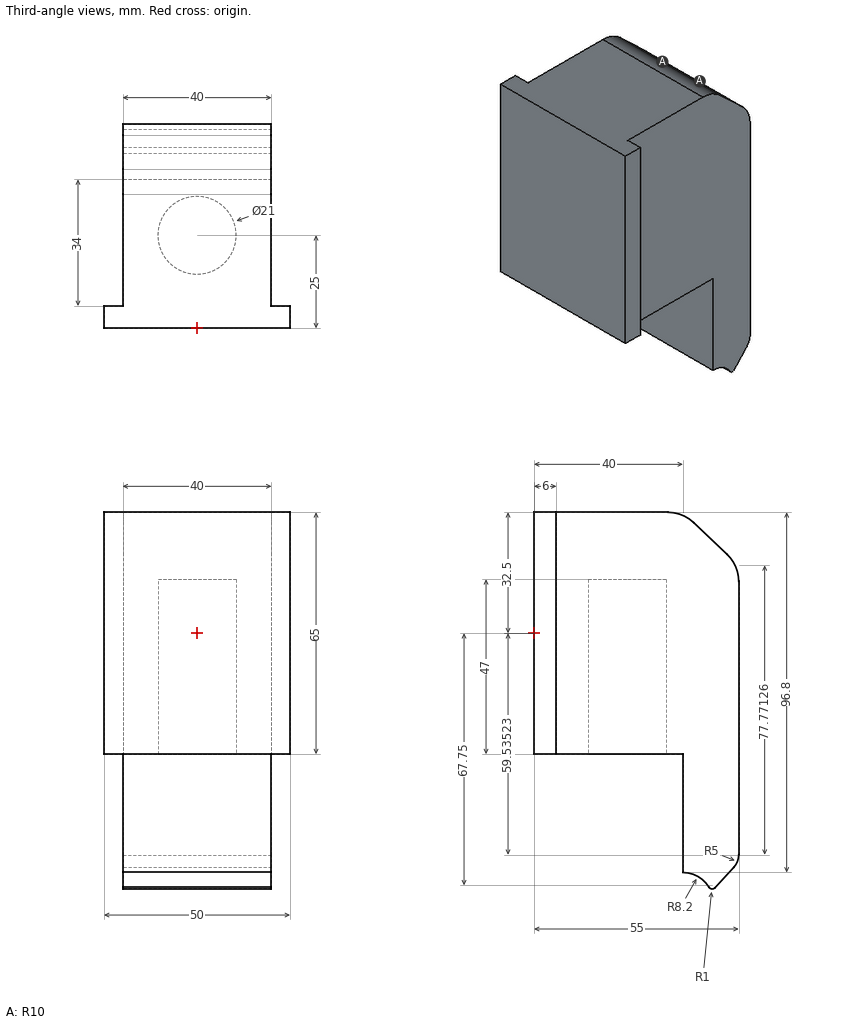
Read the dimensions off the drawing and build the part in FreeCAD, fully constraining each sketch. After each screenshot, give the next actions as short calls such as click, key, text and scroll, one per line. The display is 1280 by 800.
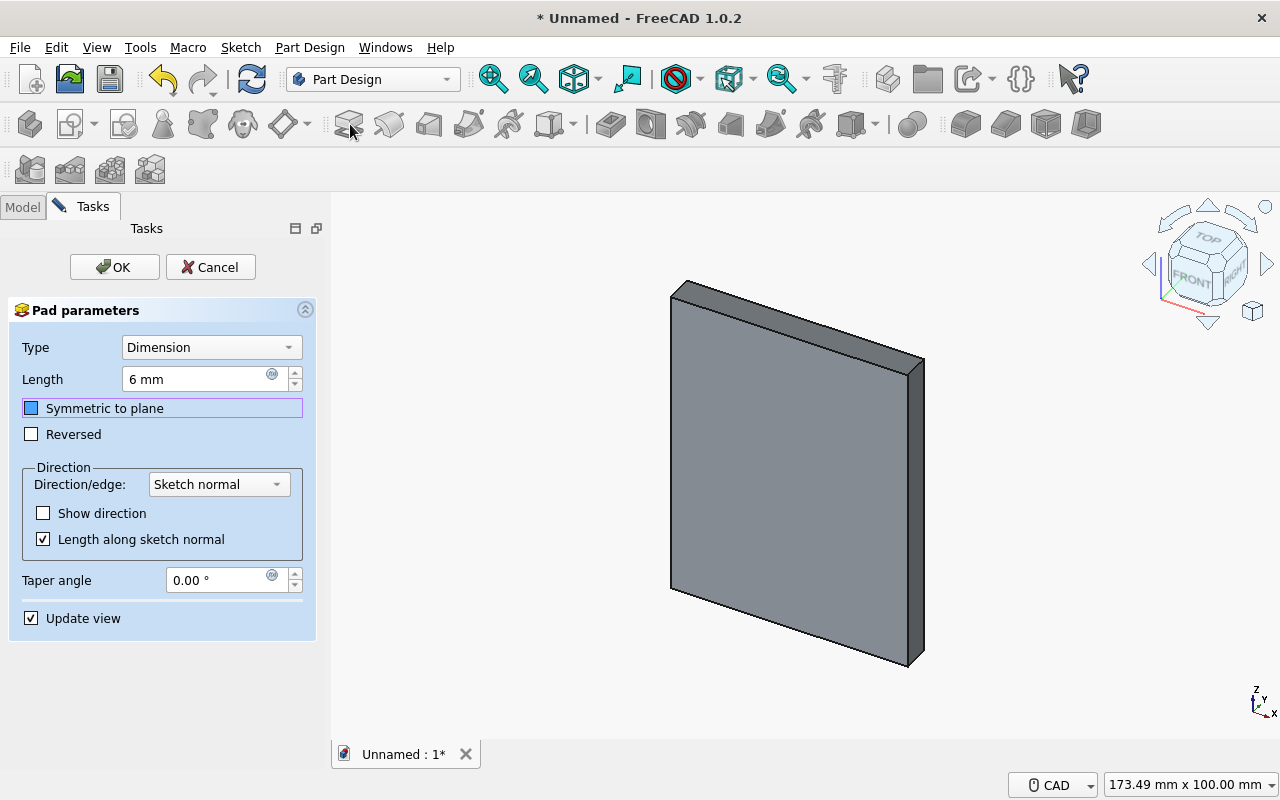
click(30, 434)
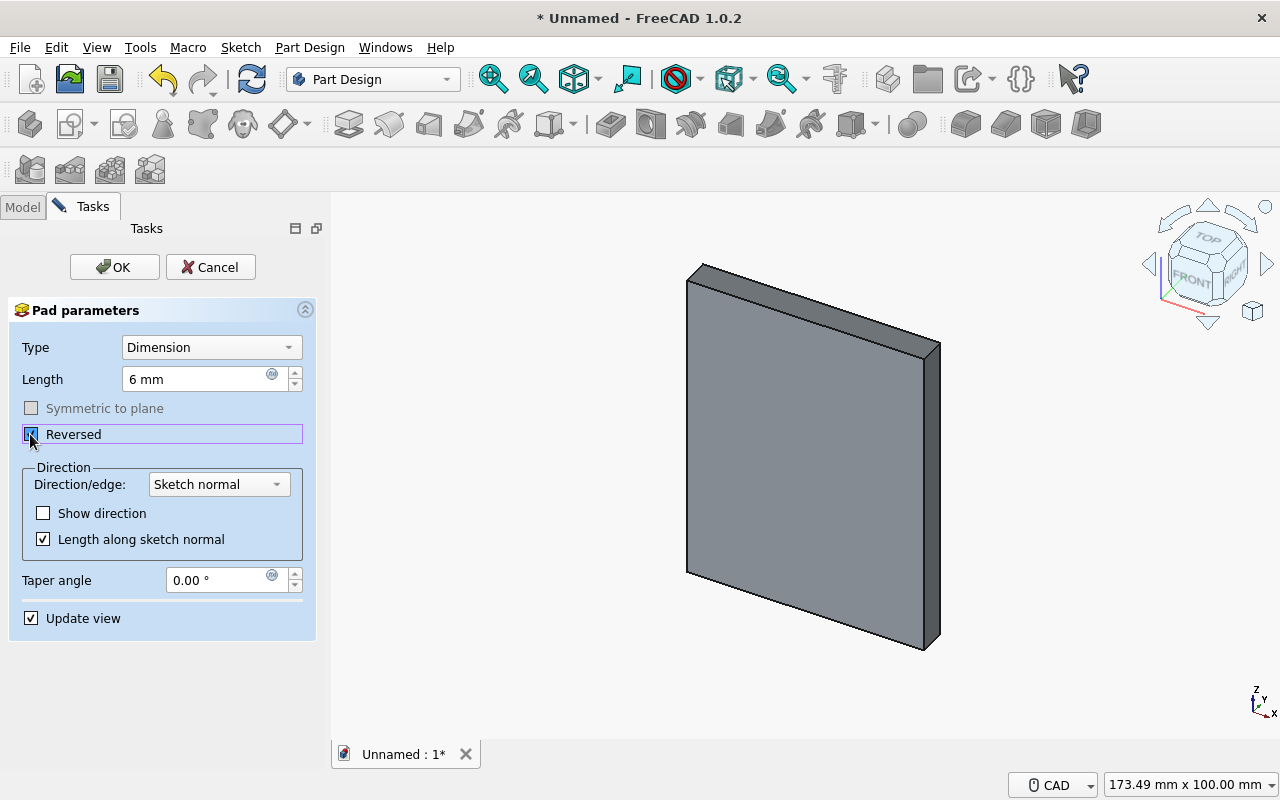
click(115, 267)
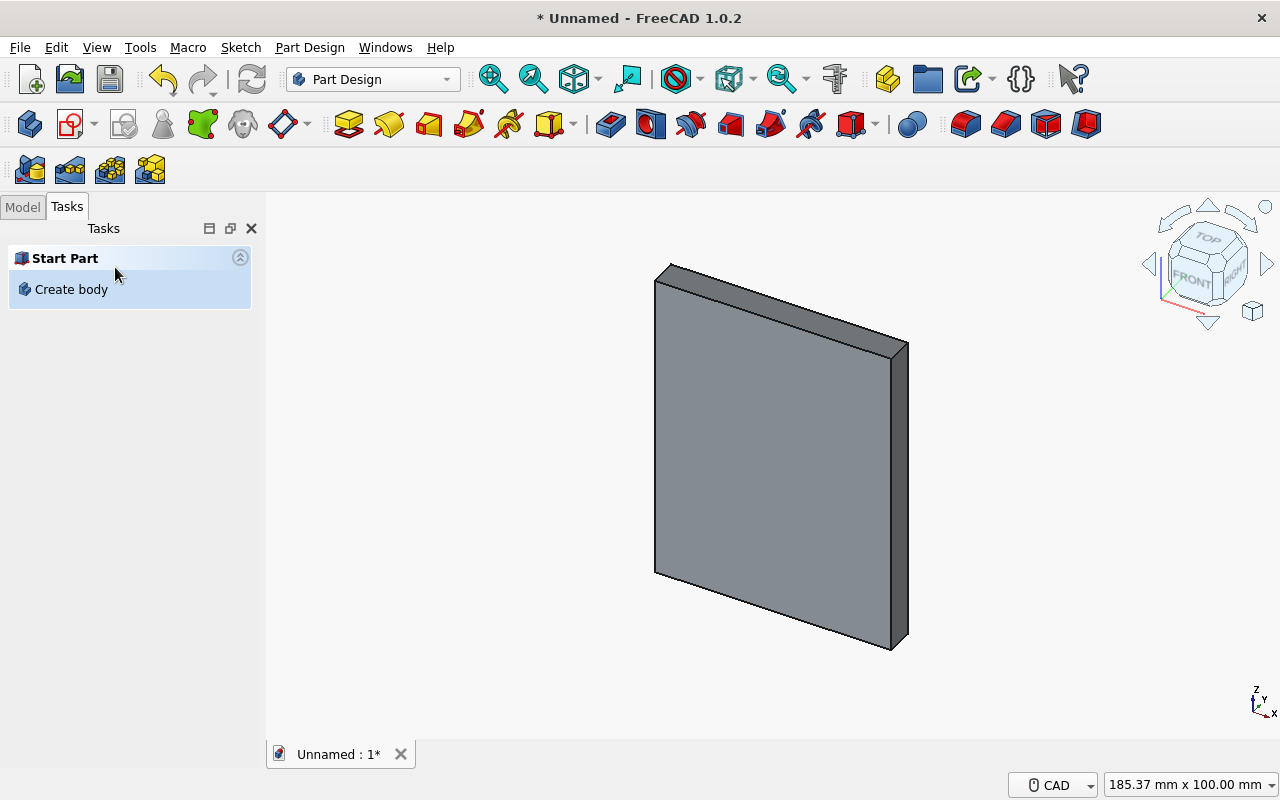
key(4)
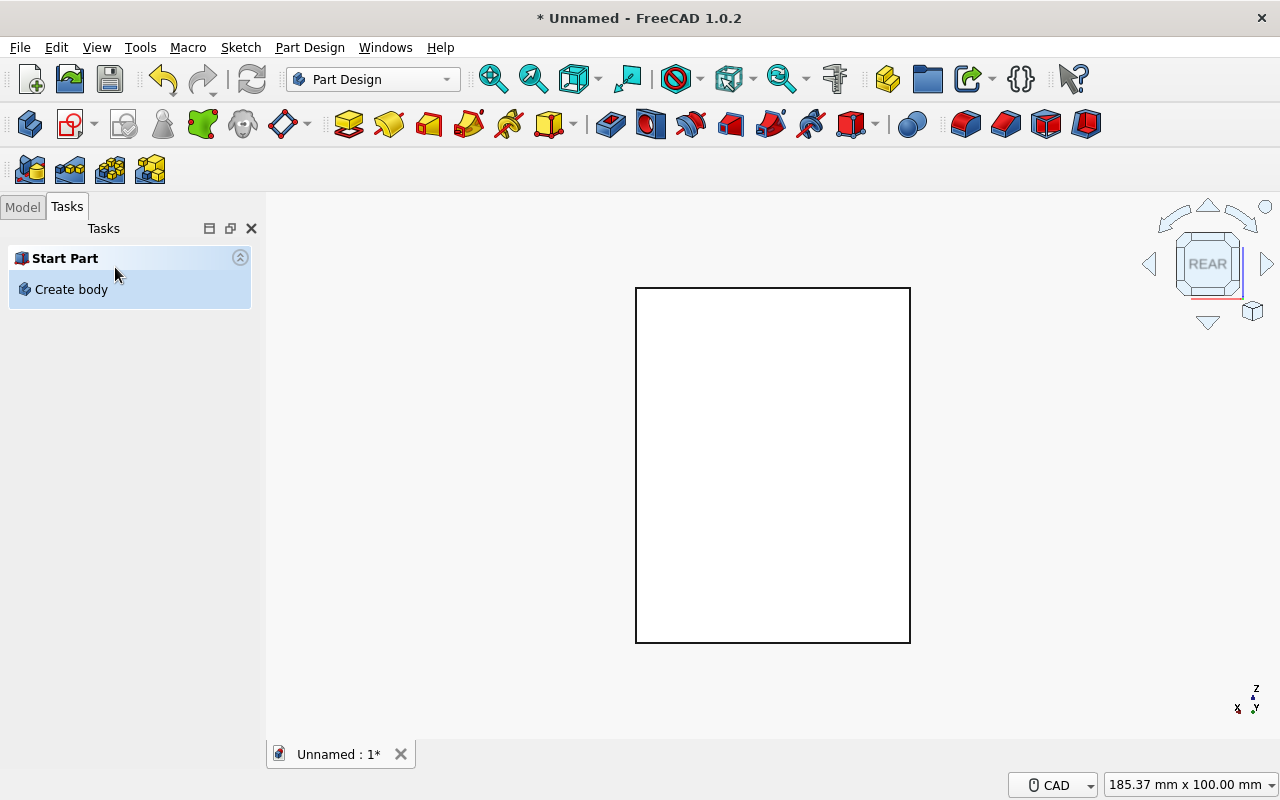
click(773, 464)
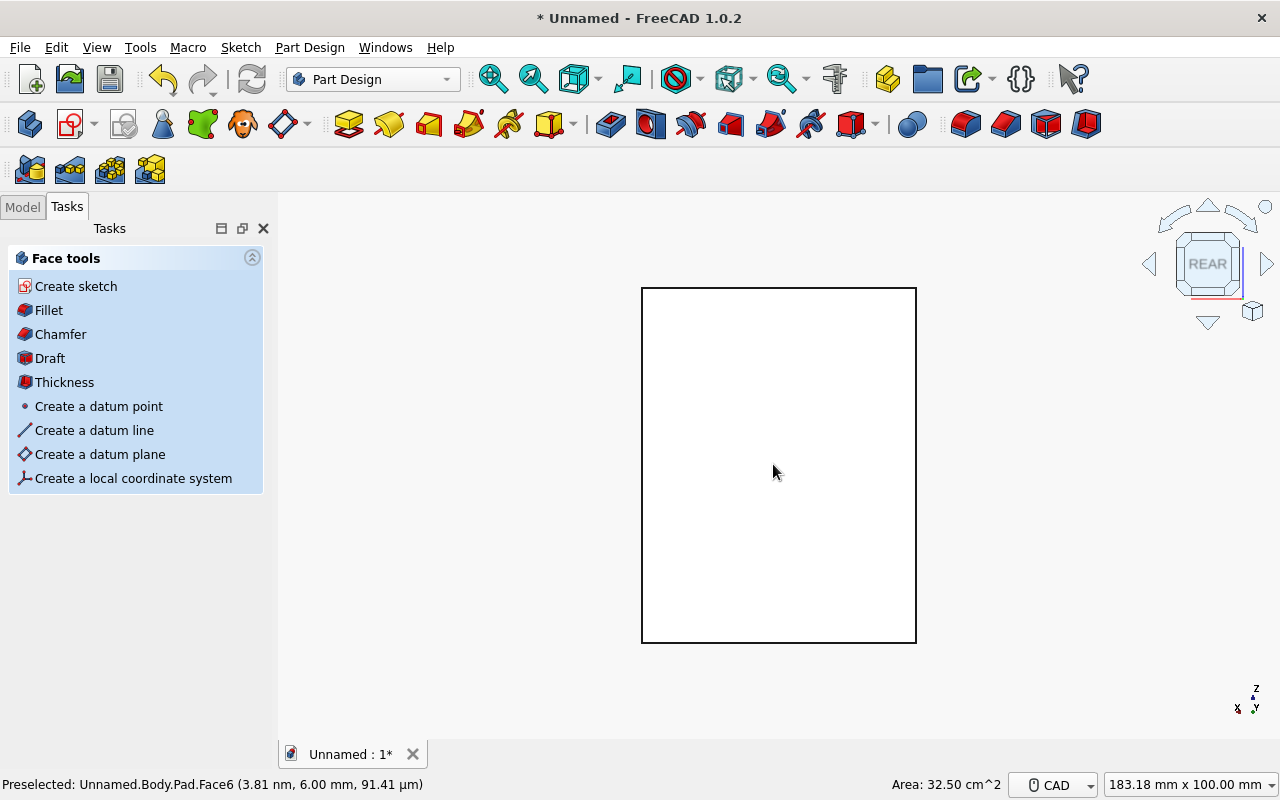
click(70, 124)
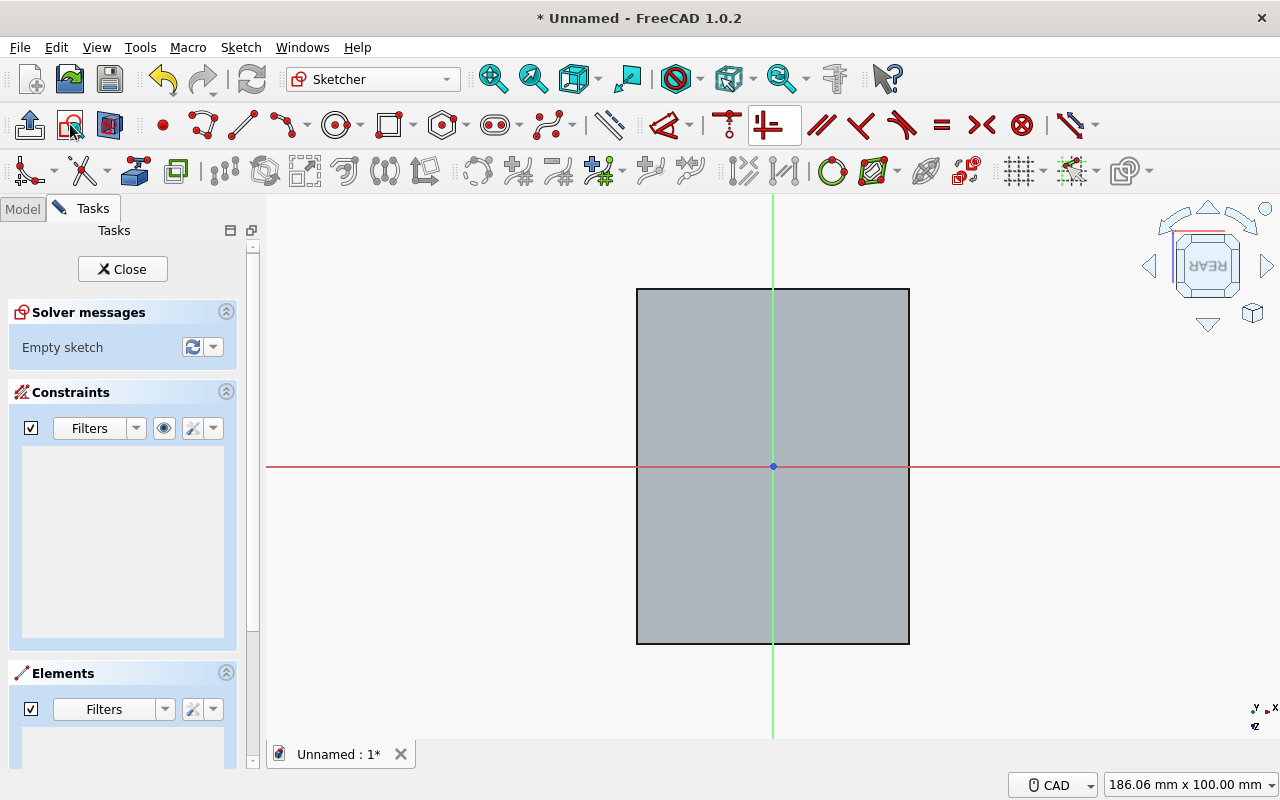
click(416, 126)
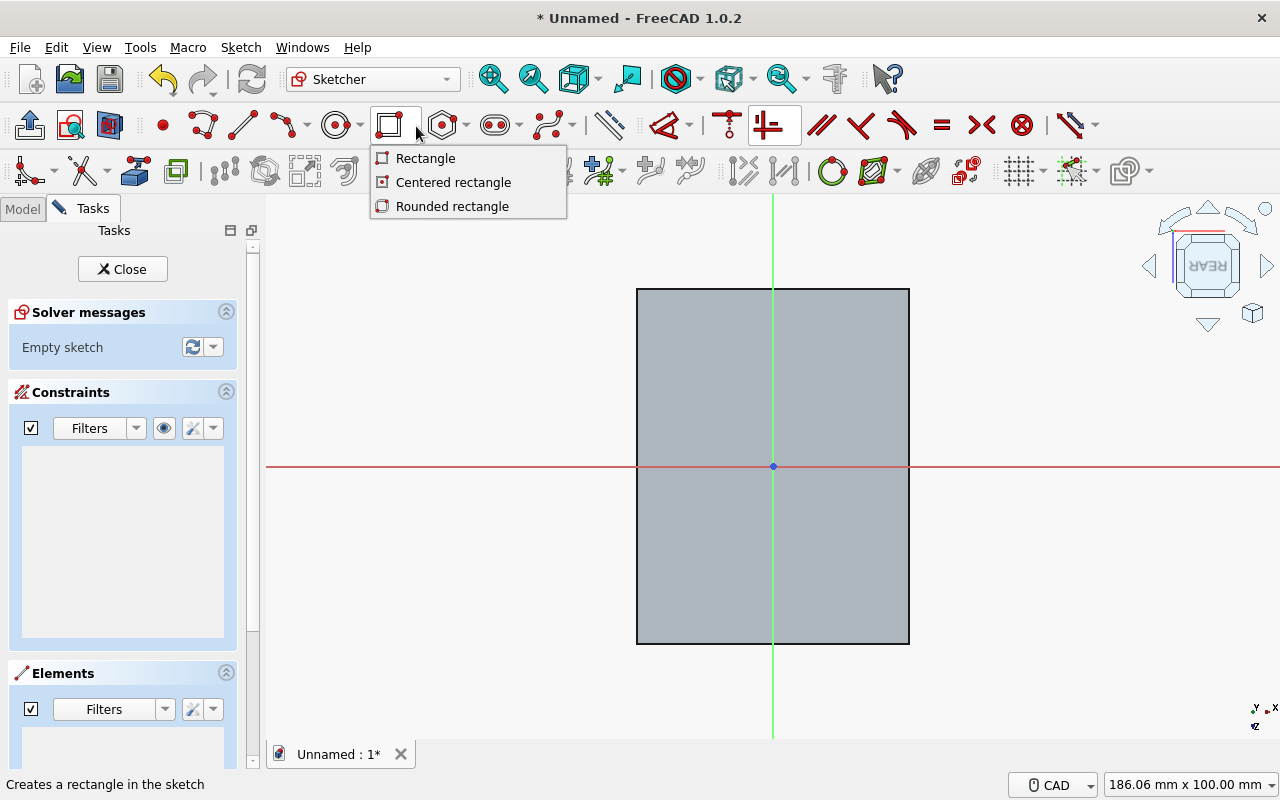
click(468, 182)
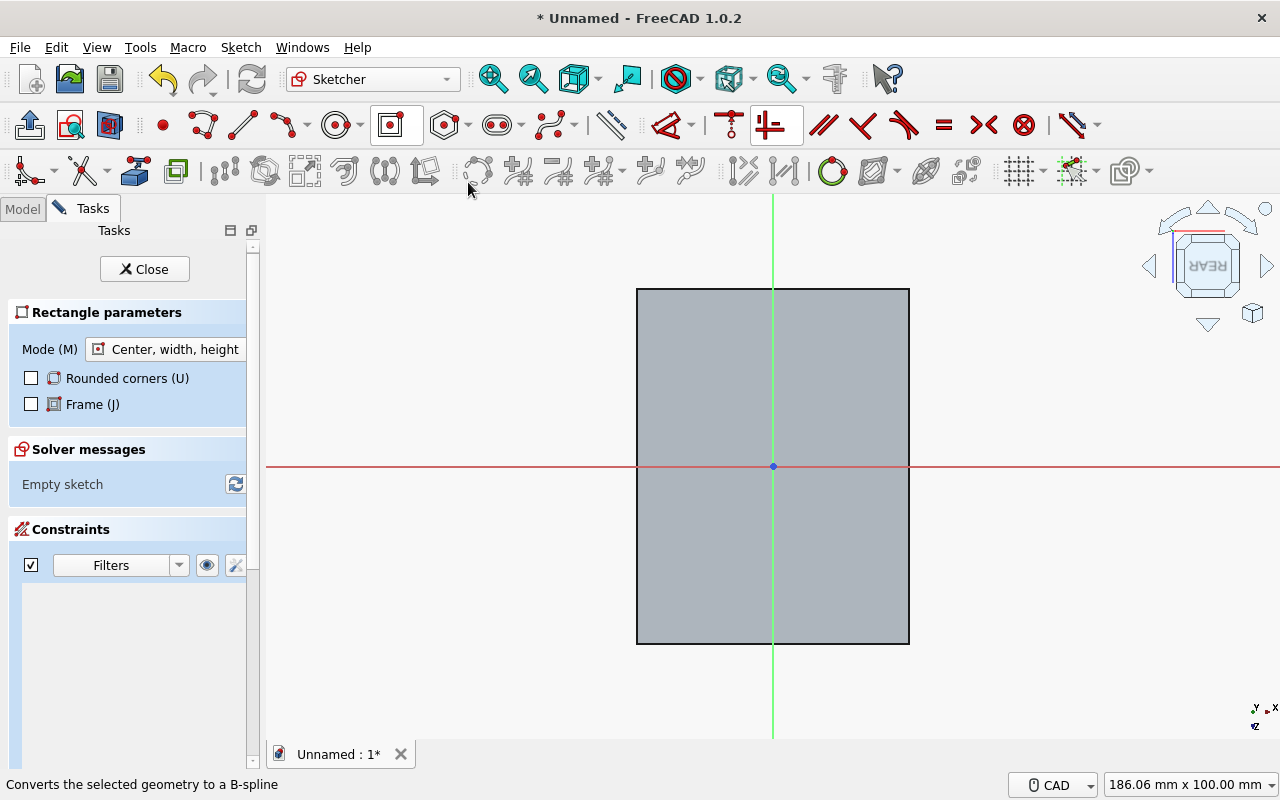
click(773, 467)
move(882, 289)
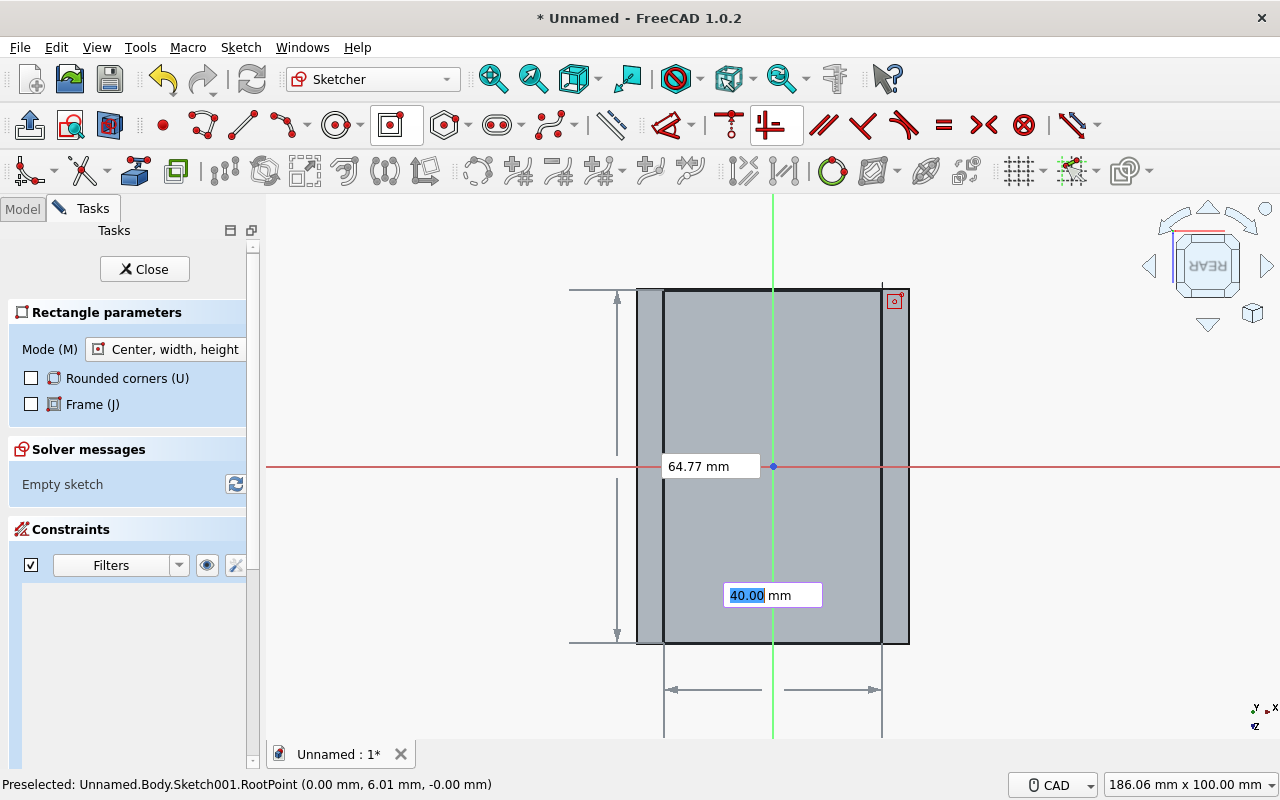
text(40)
key(Tab)
text(65)
key(Return)
key(Escape)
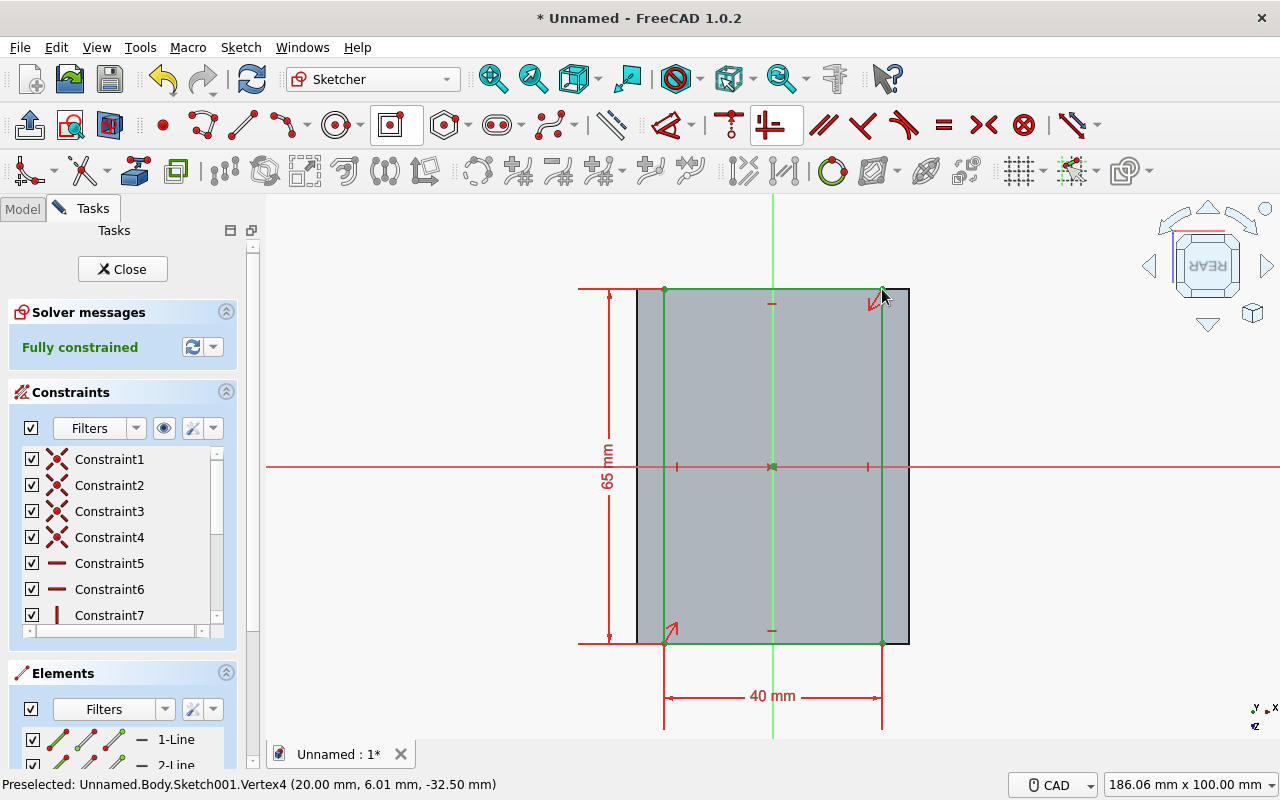
click(123, 269)